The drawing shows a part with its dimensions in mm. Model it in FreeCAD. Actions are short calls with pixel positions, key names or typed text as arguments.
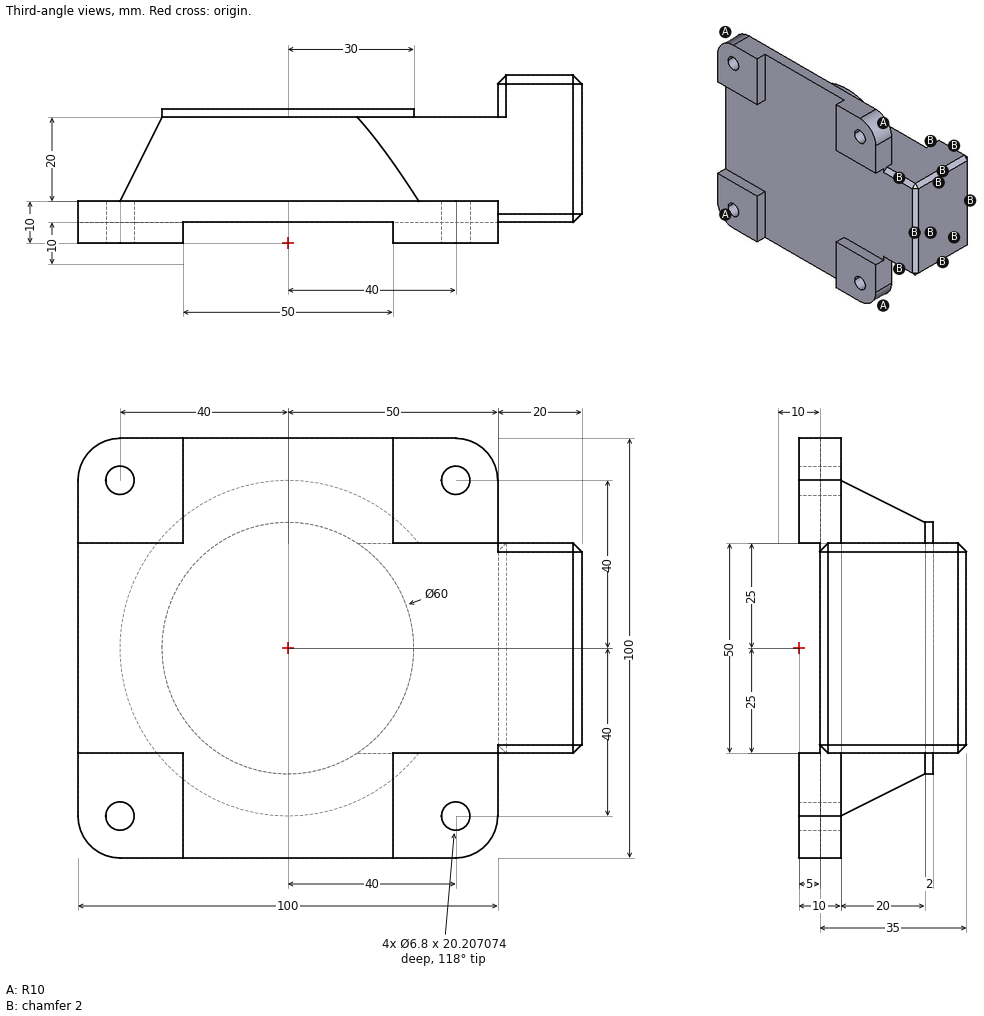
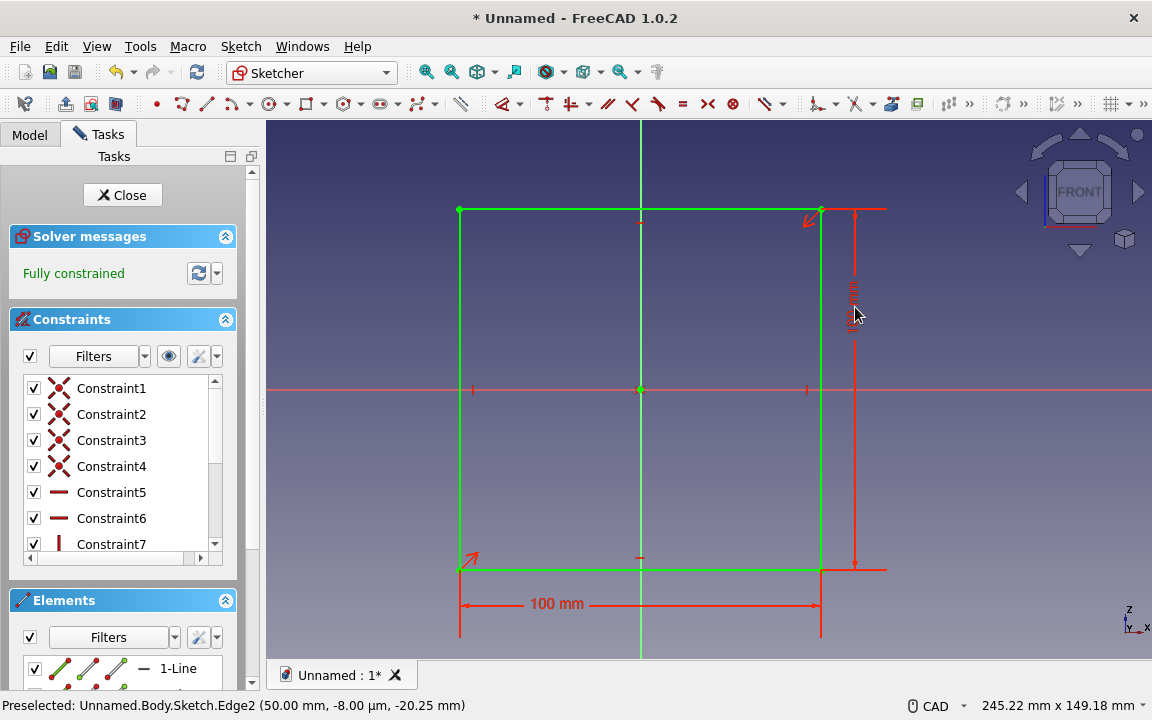
click(123, 195)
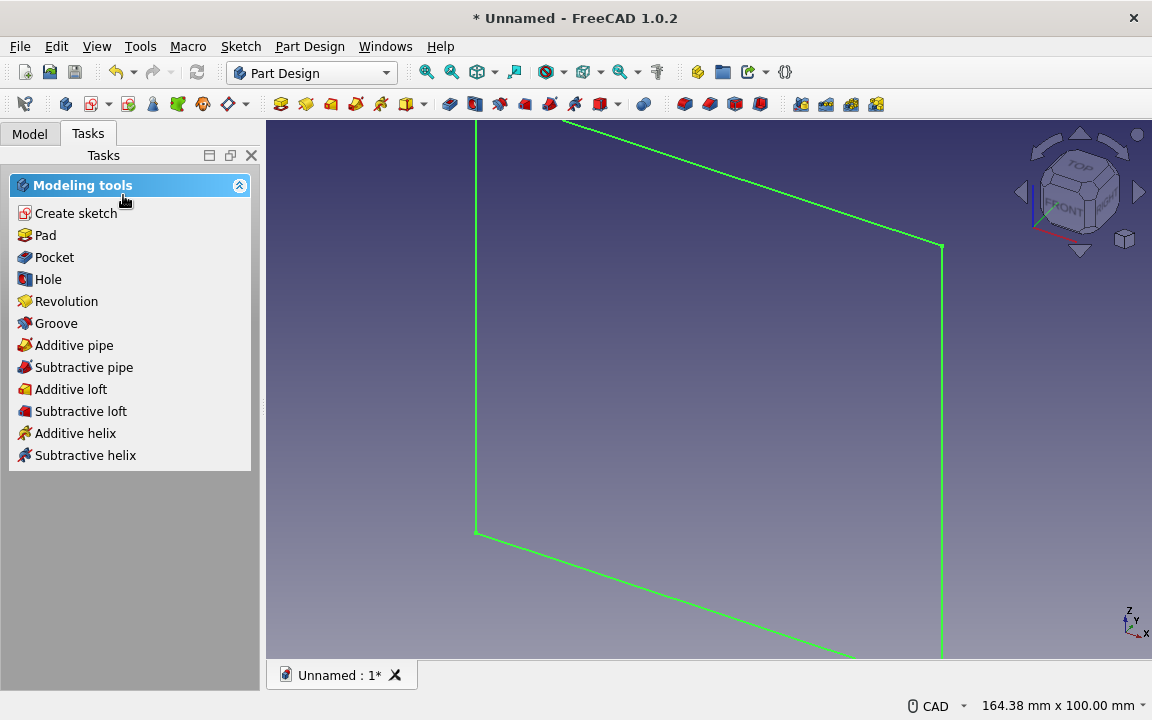
click(281, 104)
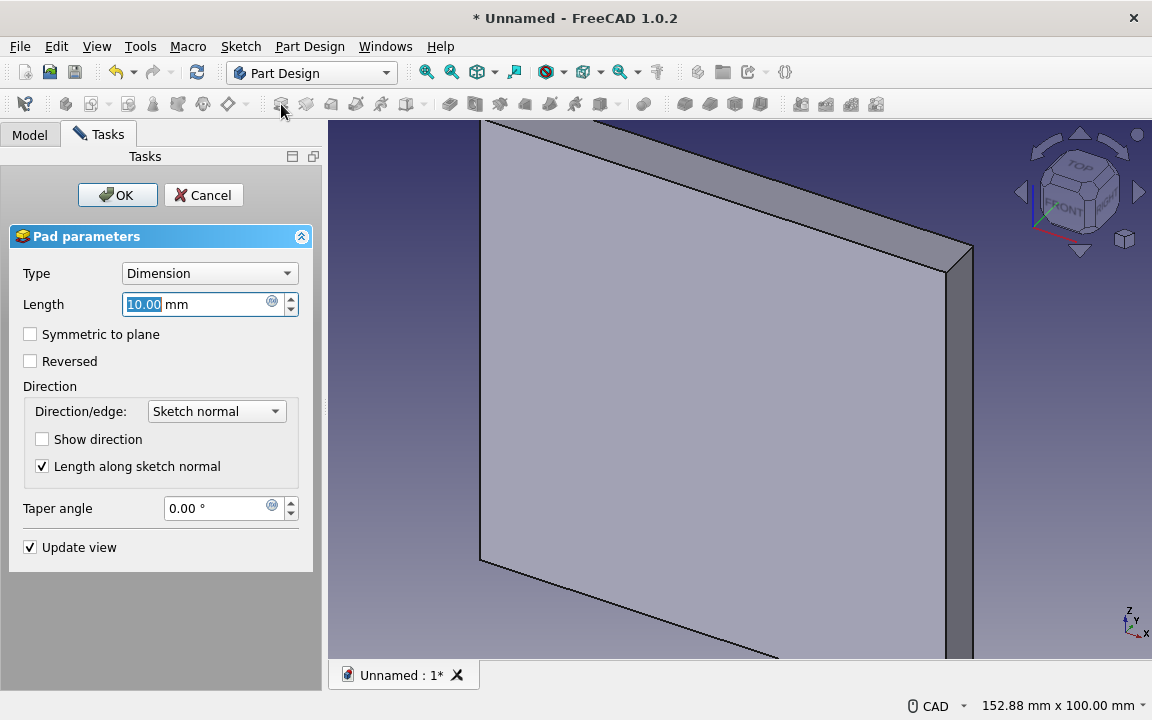
text(10)
key(Tab)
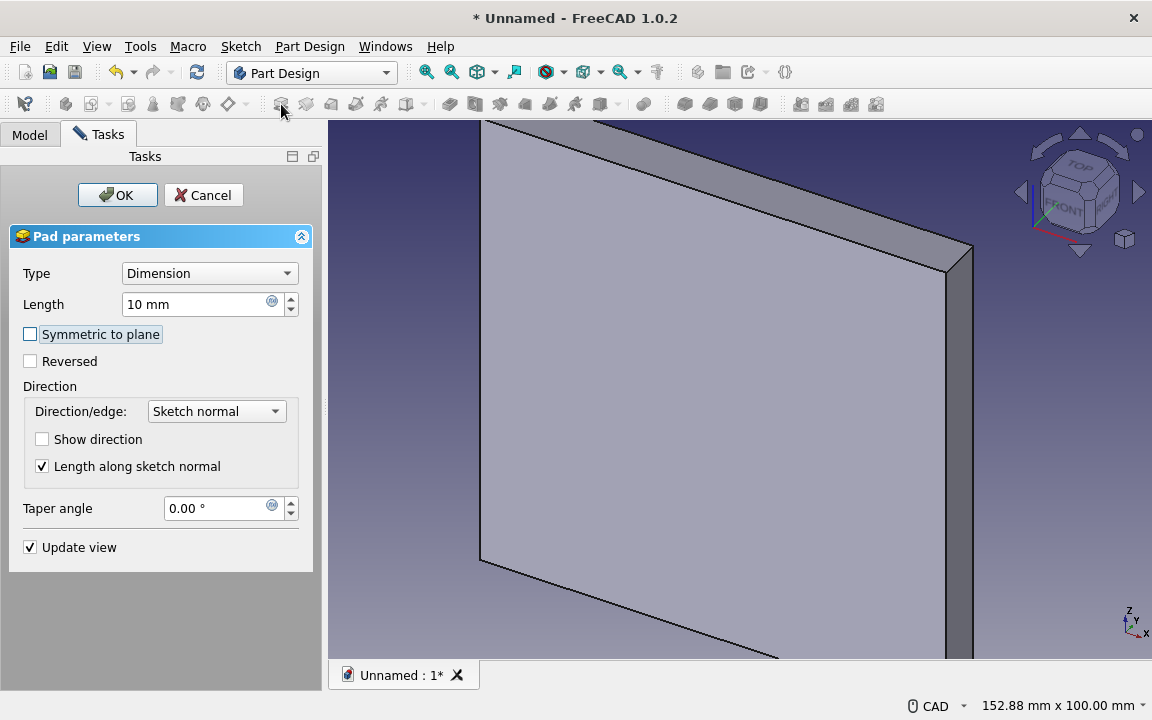
click(31, 361)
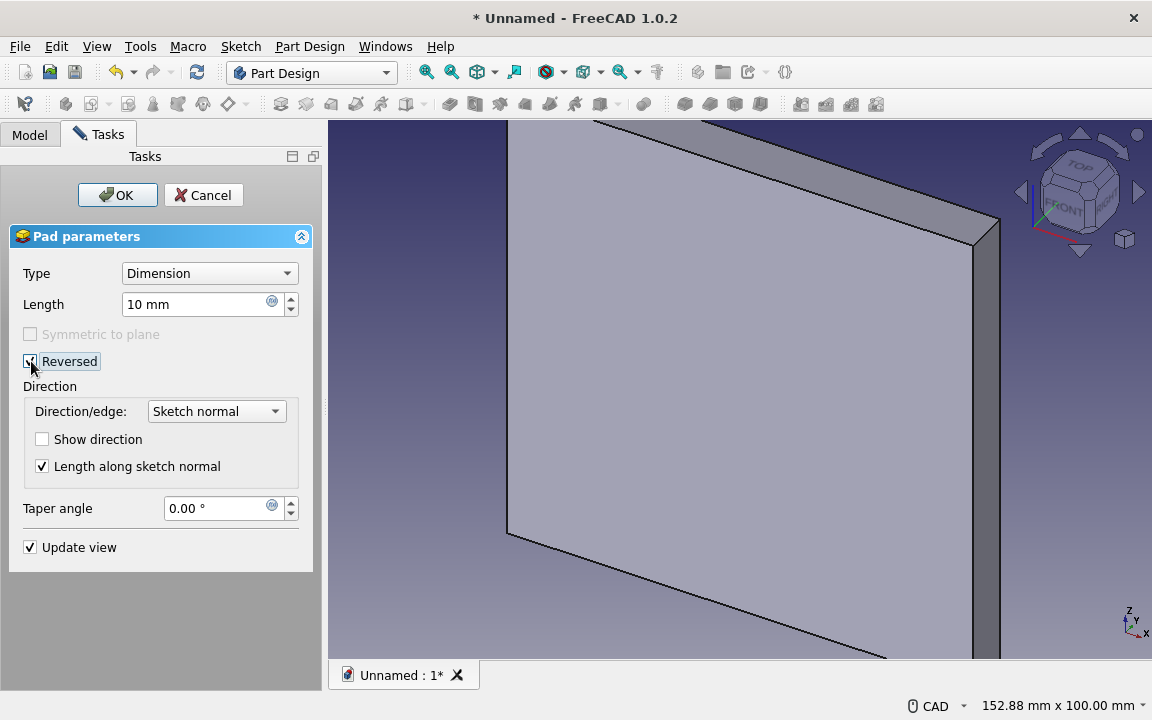
click(118, 195)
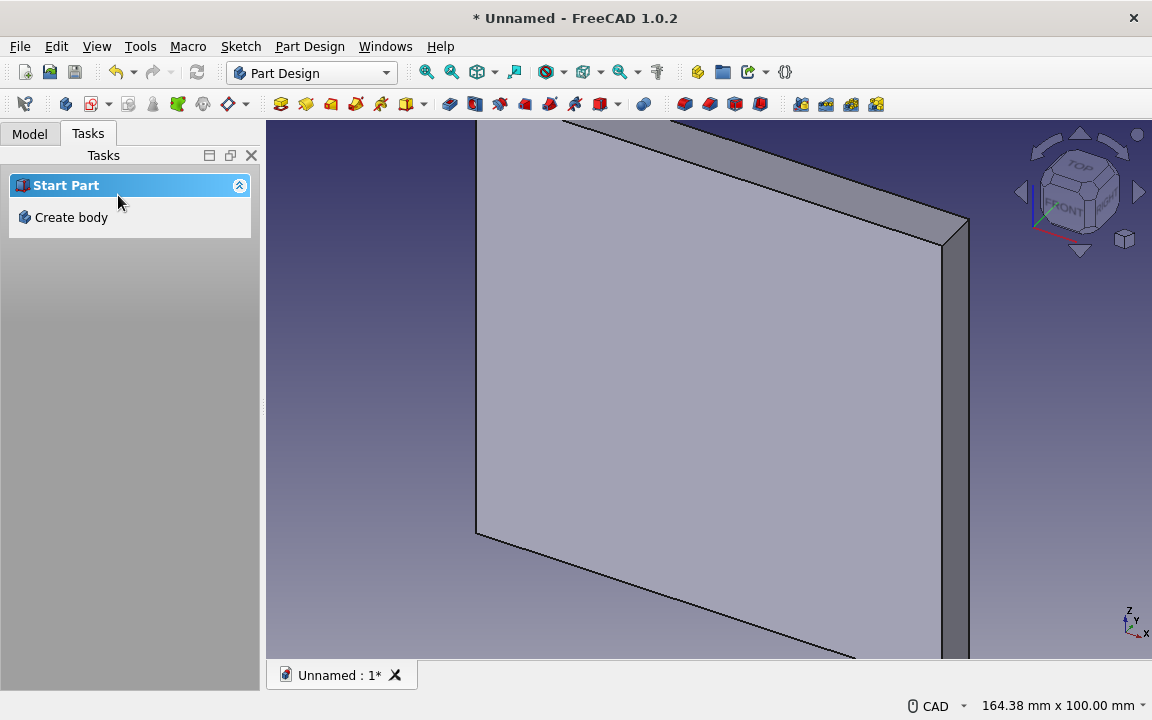
key(v)
key(f)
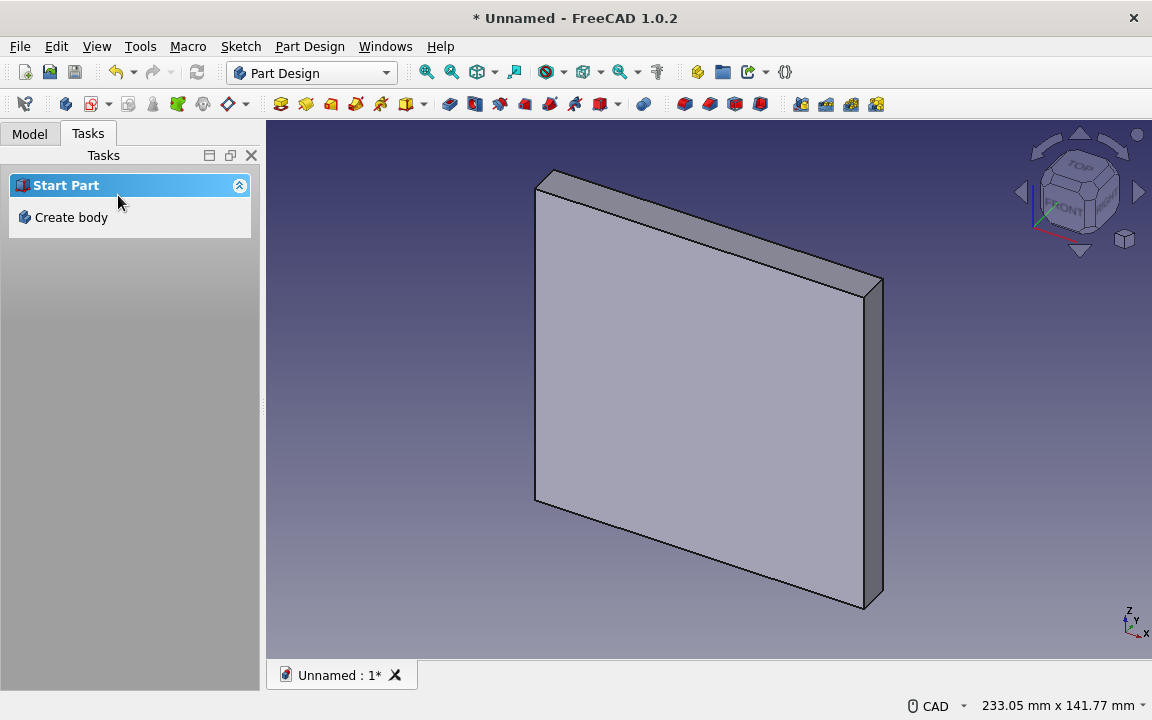
click(850, 280)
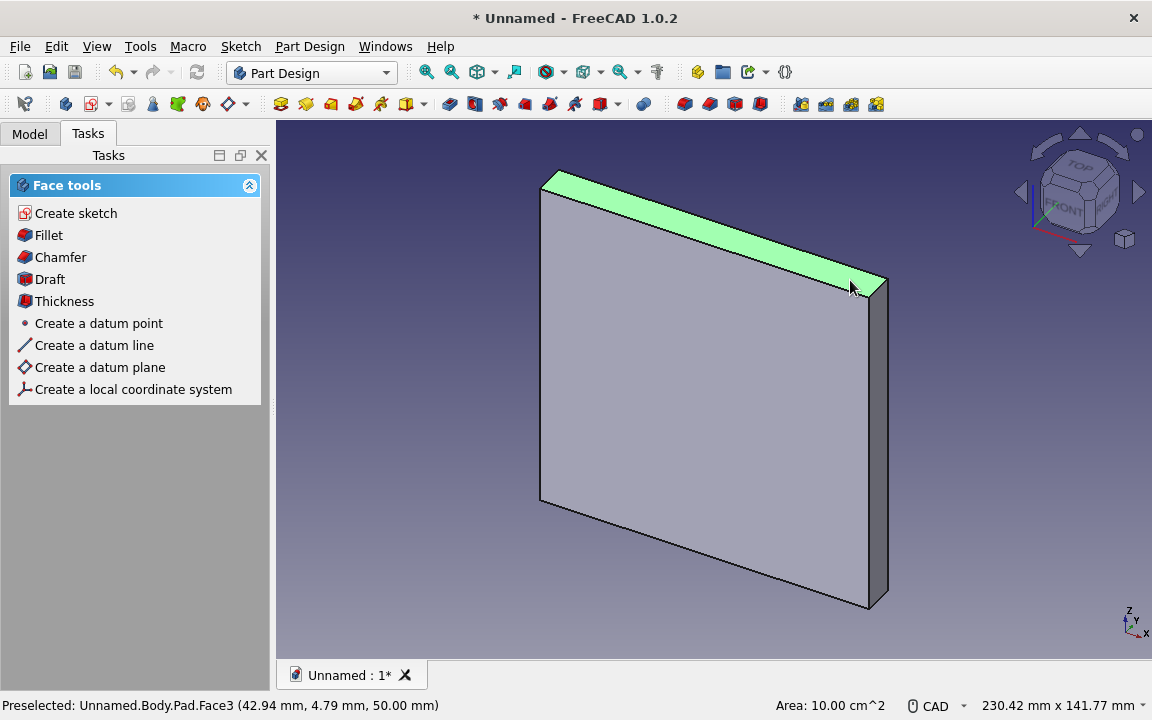
click(90, 104)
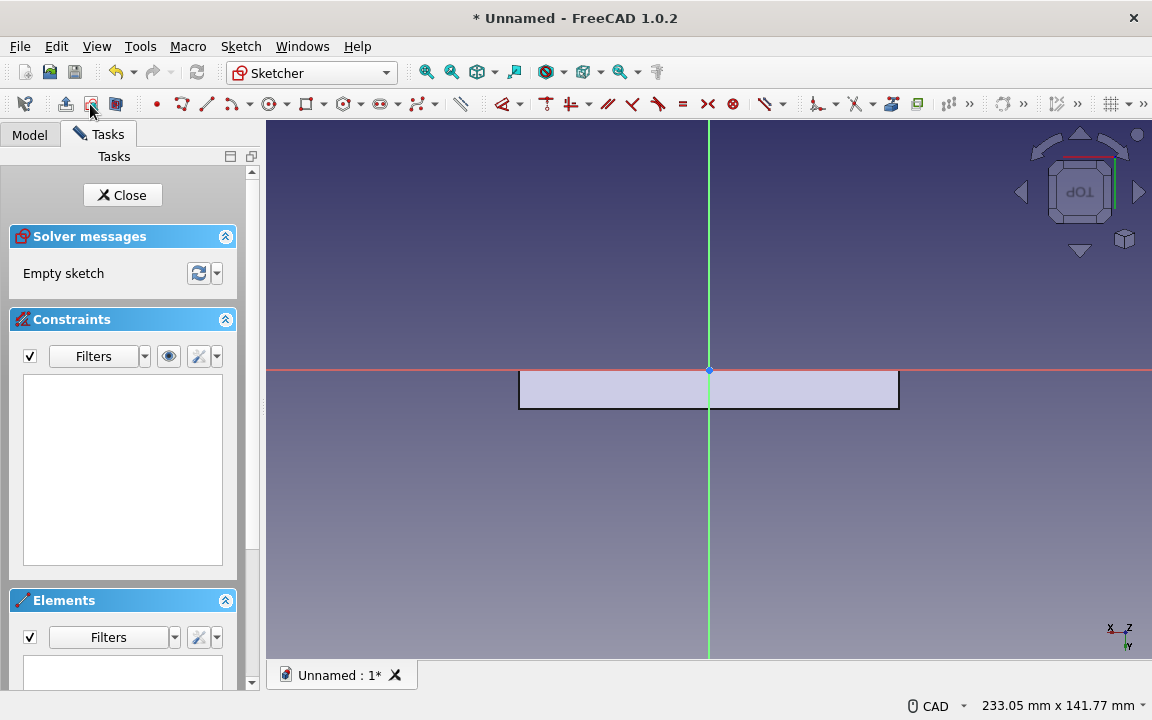
scroll(749, 359, up, 5)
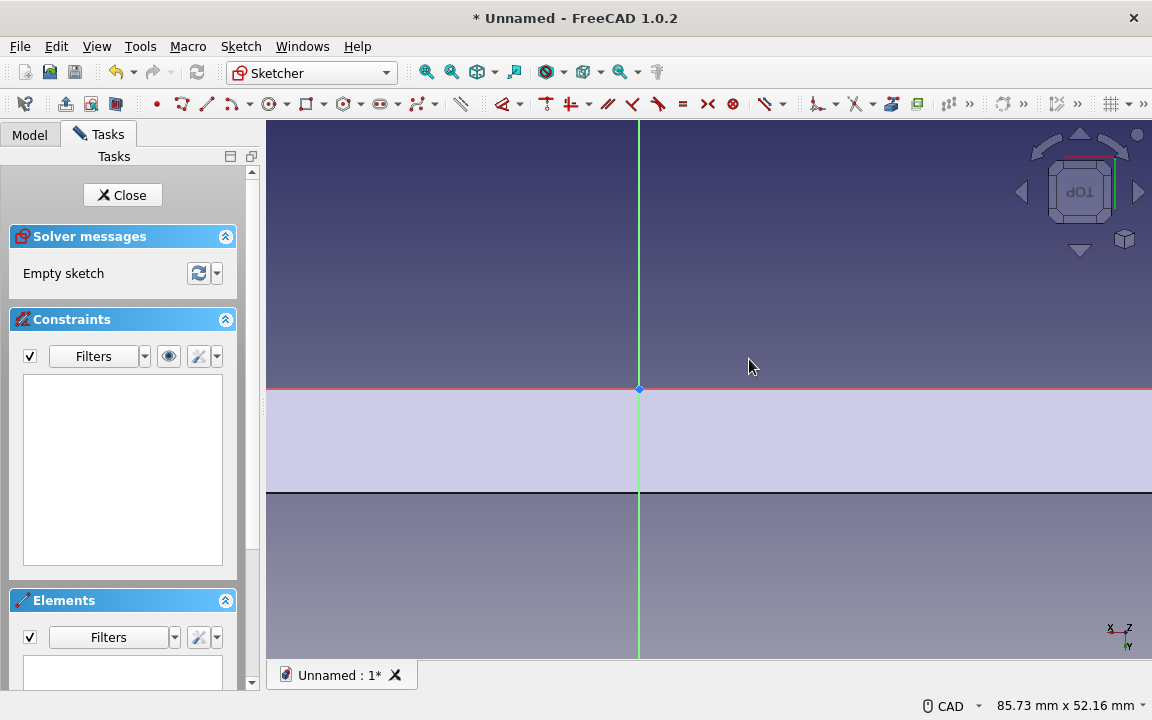
key(g)
key(v)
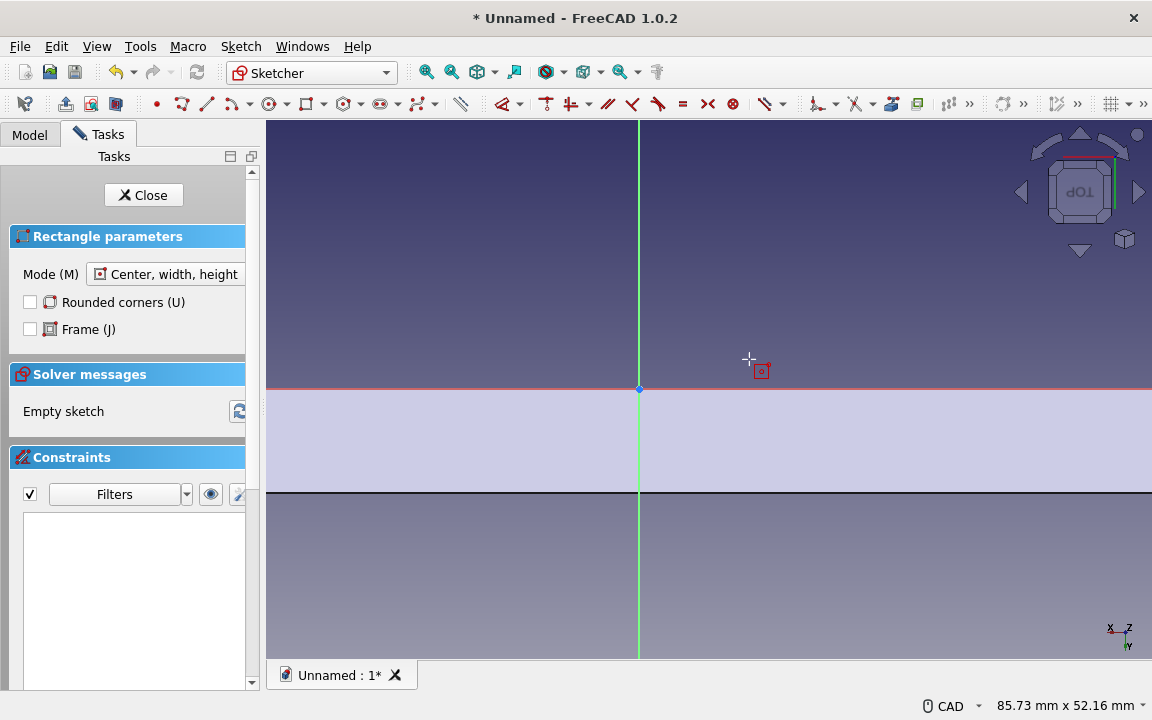
click(639, 389)
click(898, 338)
key(Escape)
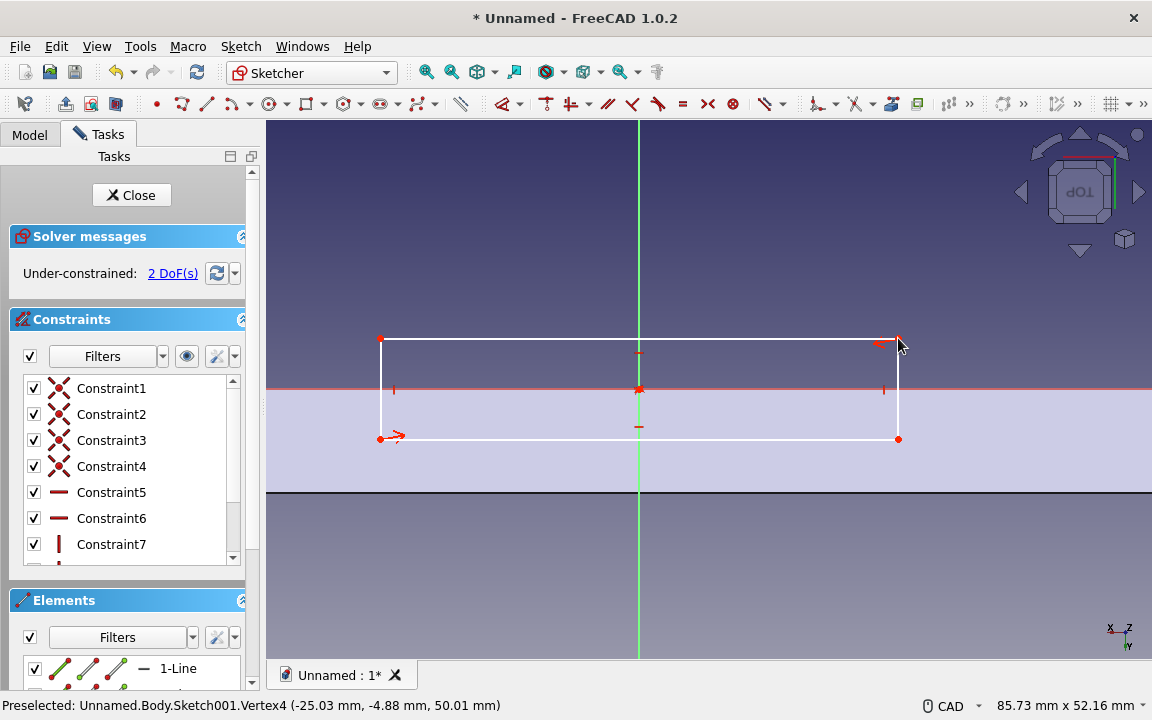
click(502, 104)